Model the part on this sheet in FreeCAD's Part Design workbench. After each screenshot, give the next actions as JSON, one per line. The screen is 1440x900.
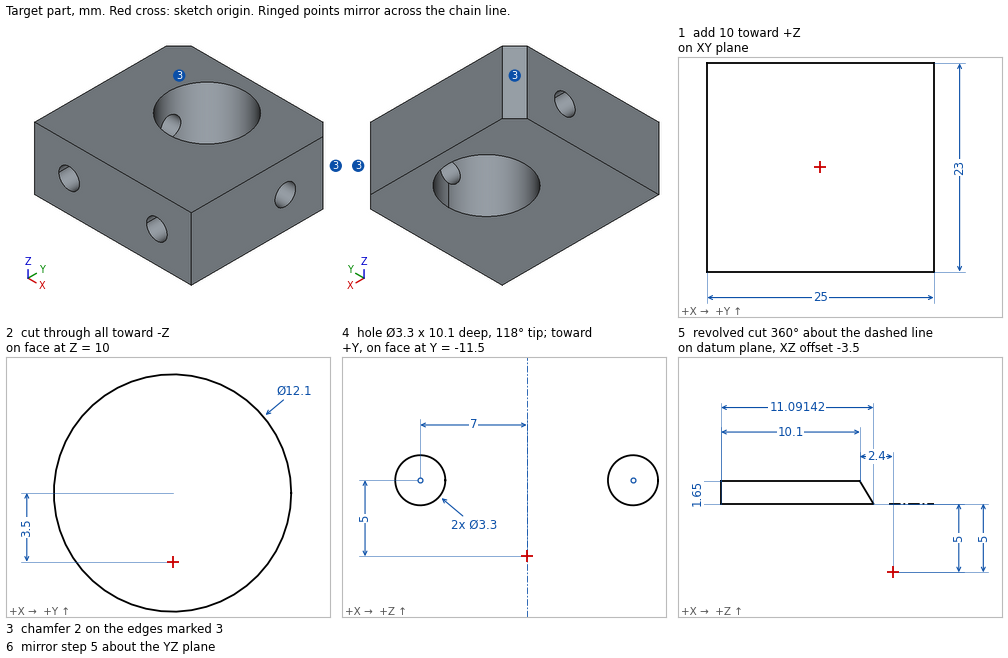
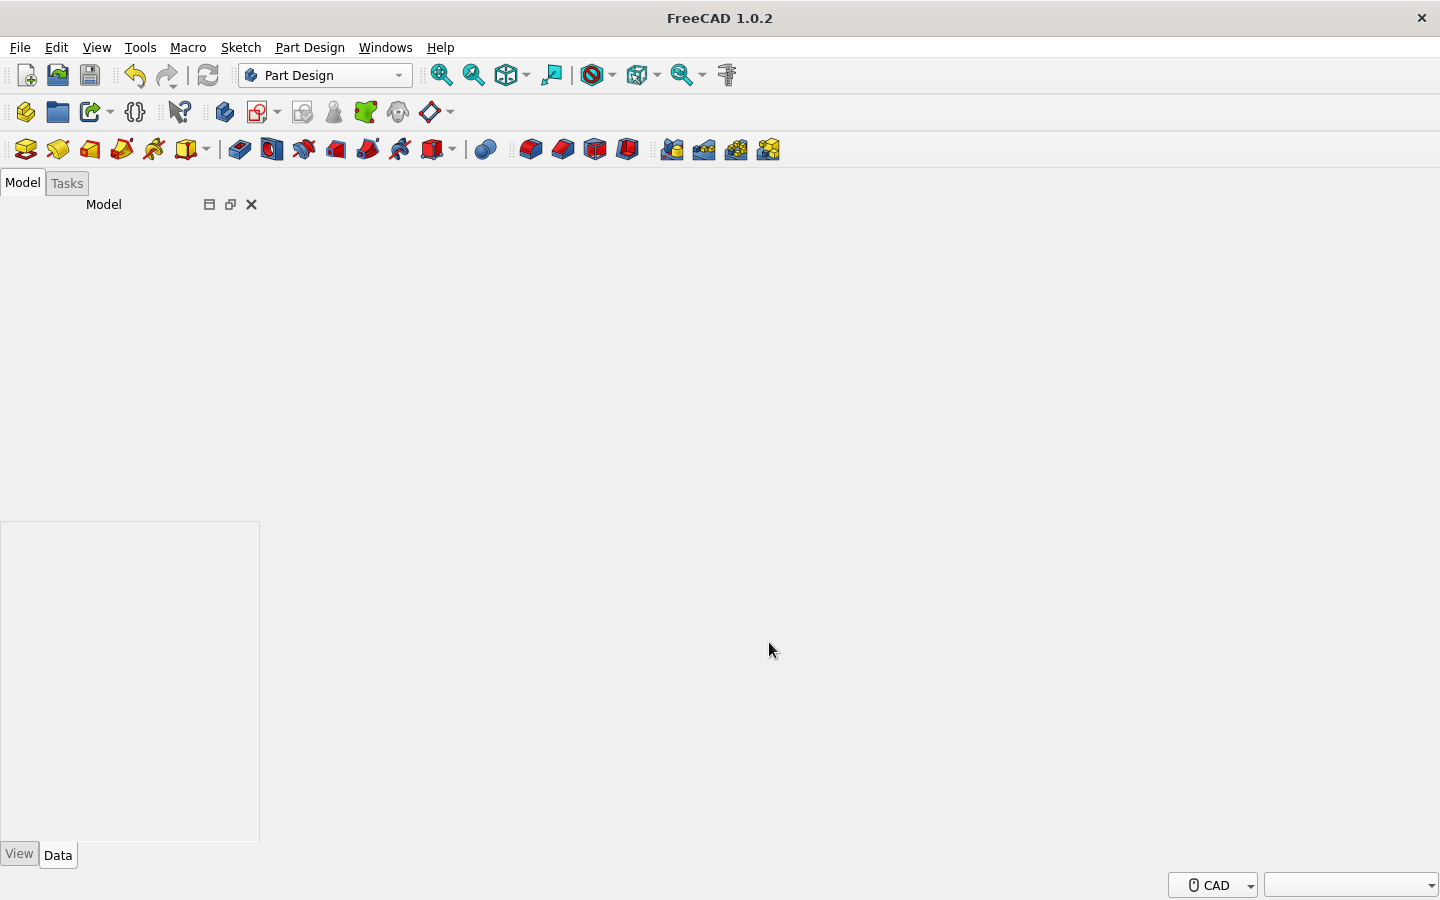
{"action": "left_click", "coordinate": [26, 76]}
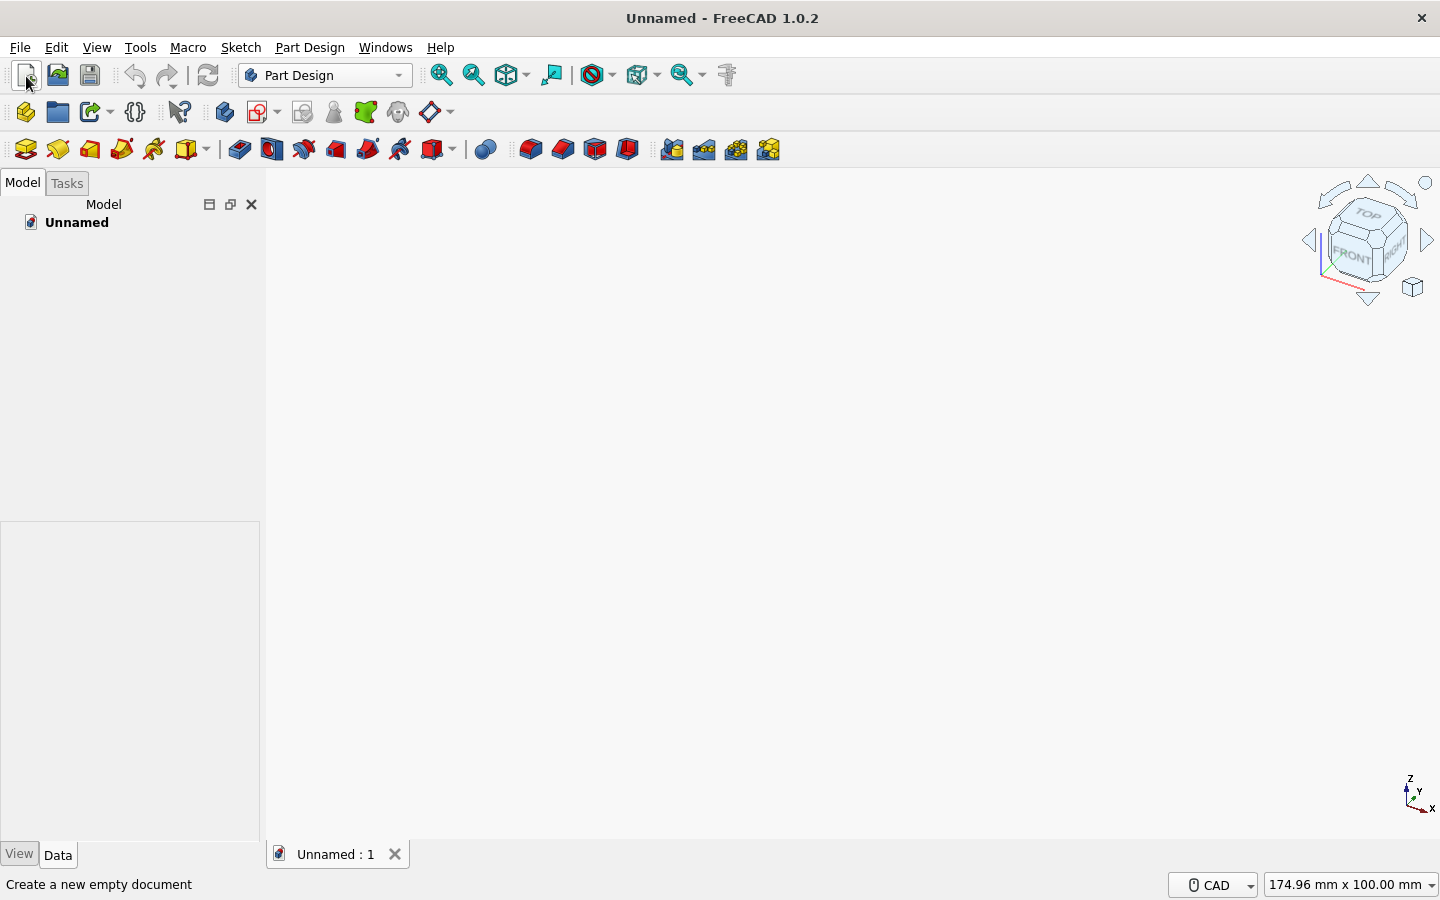
{"action": "left_click", "coordinate": [258, 112]}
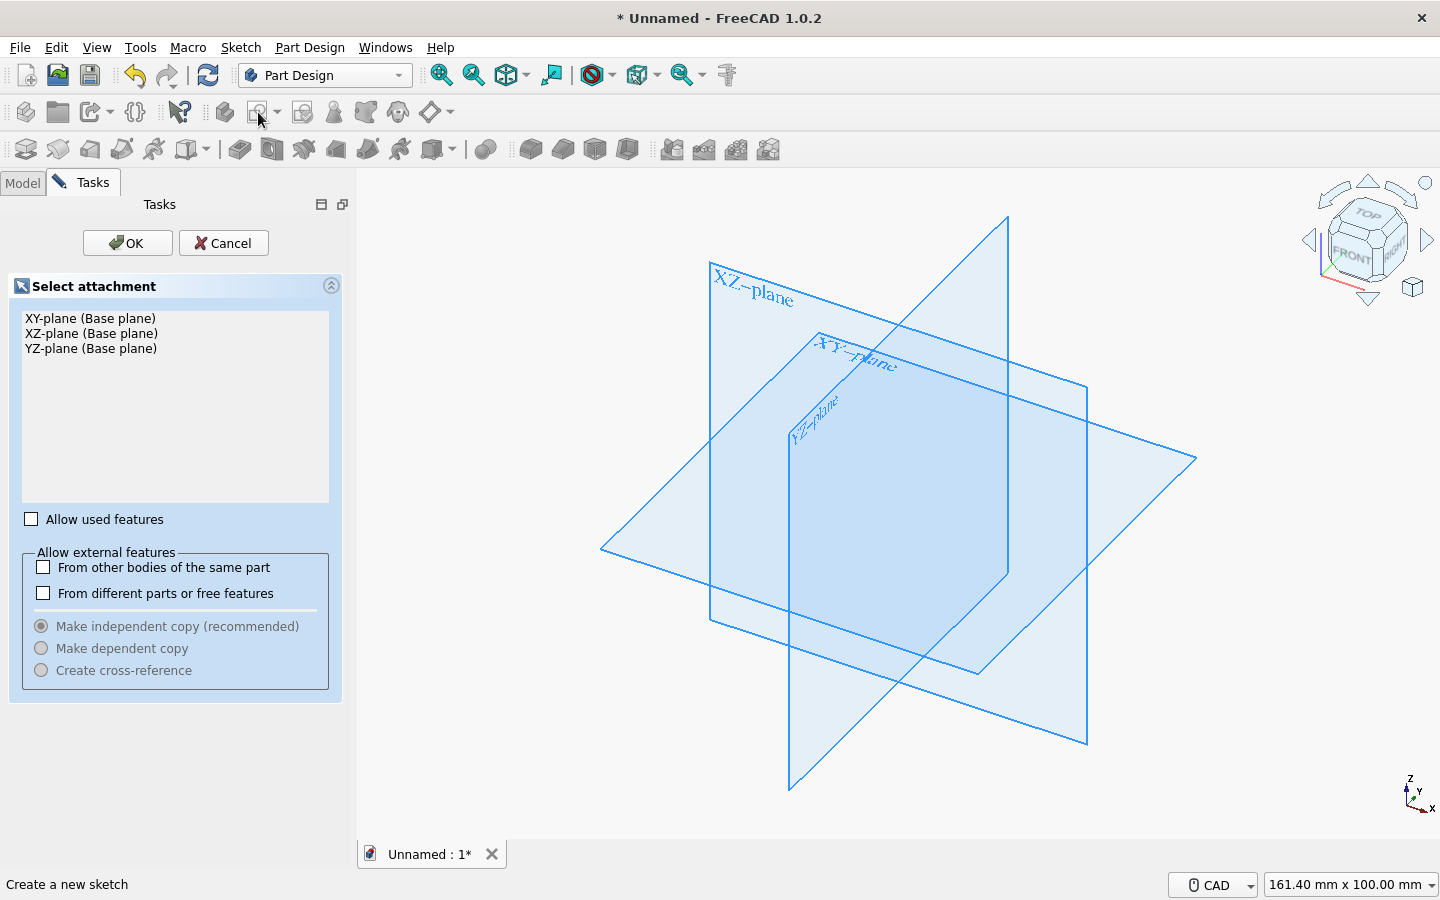
{"action": "left_click", "coordinate": [82, 318]}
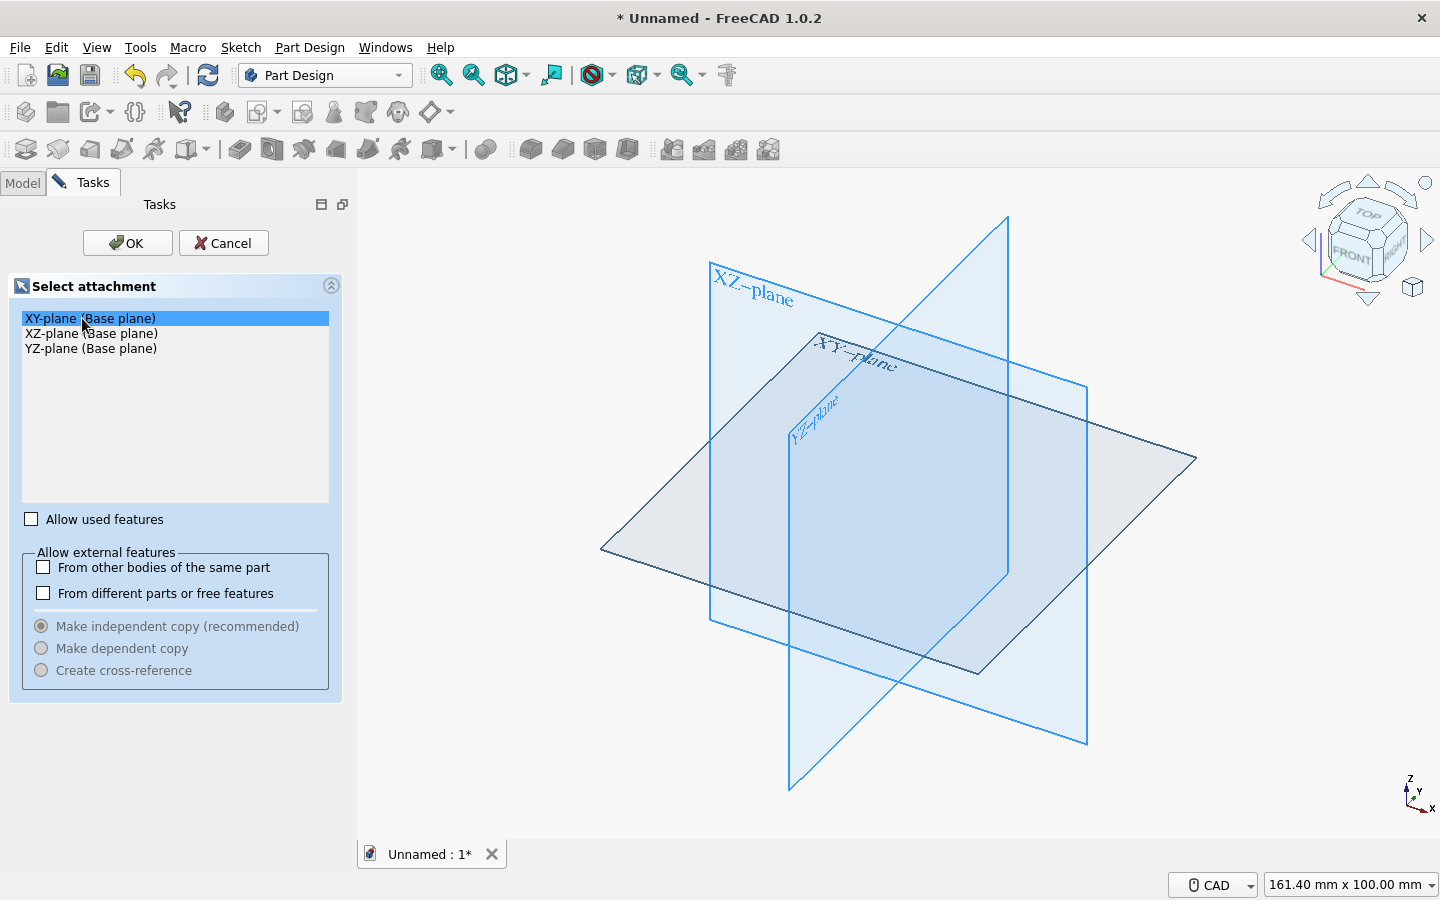
{"action": "left_click", "coordinate": [128, 243]}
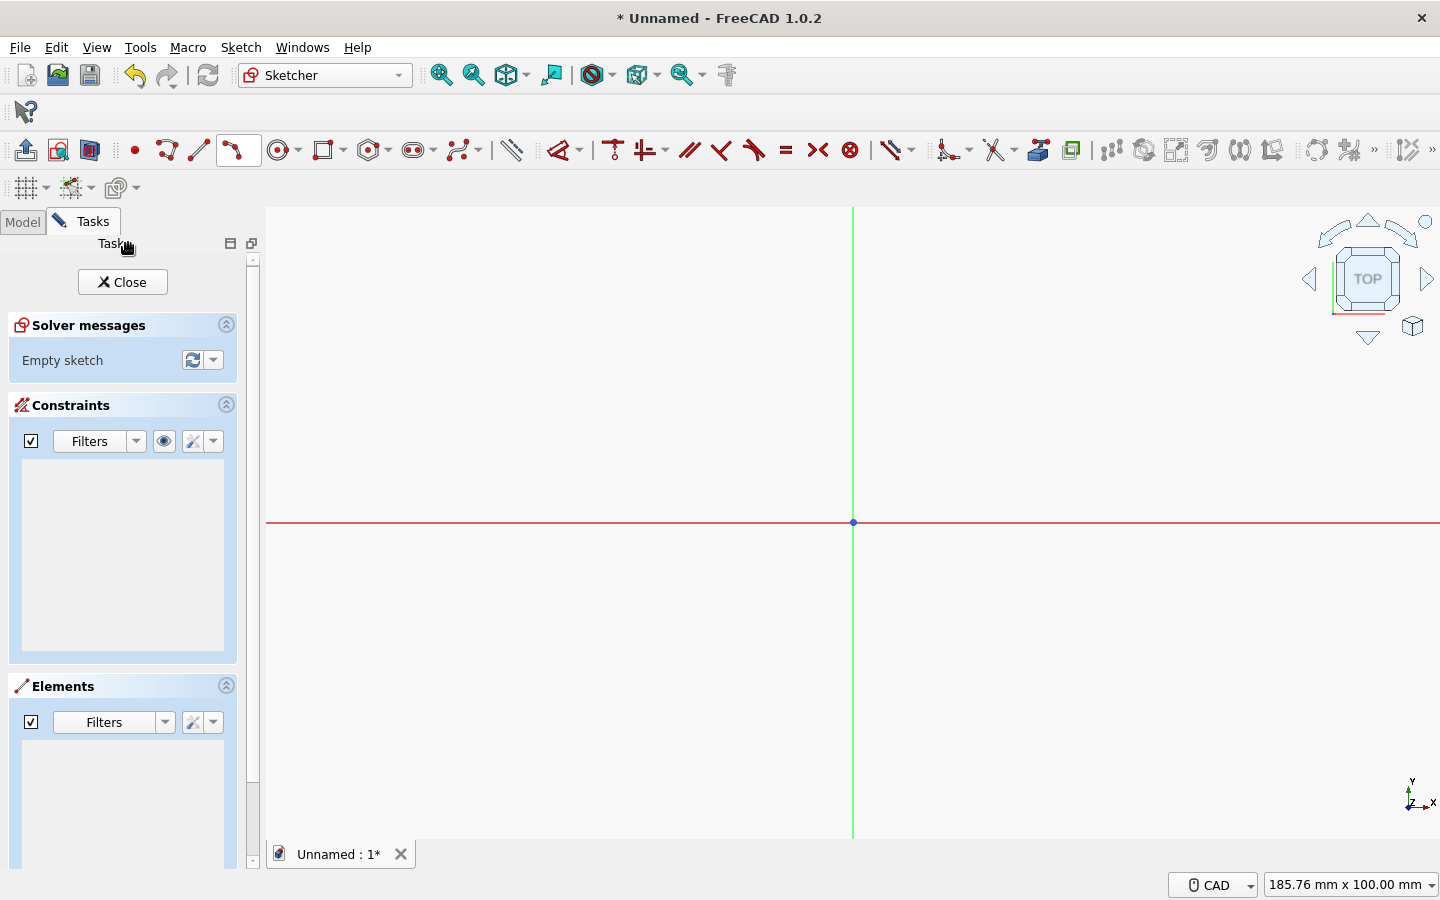
{"action": "scroll", "coordinate": [893, 523], "scroll_direction": "up", "scroll_amount": 5}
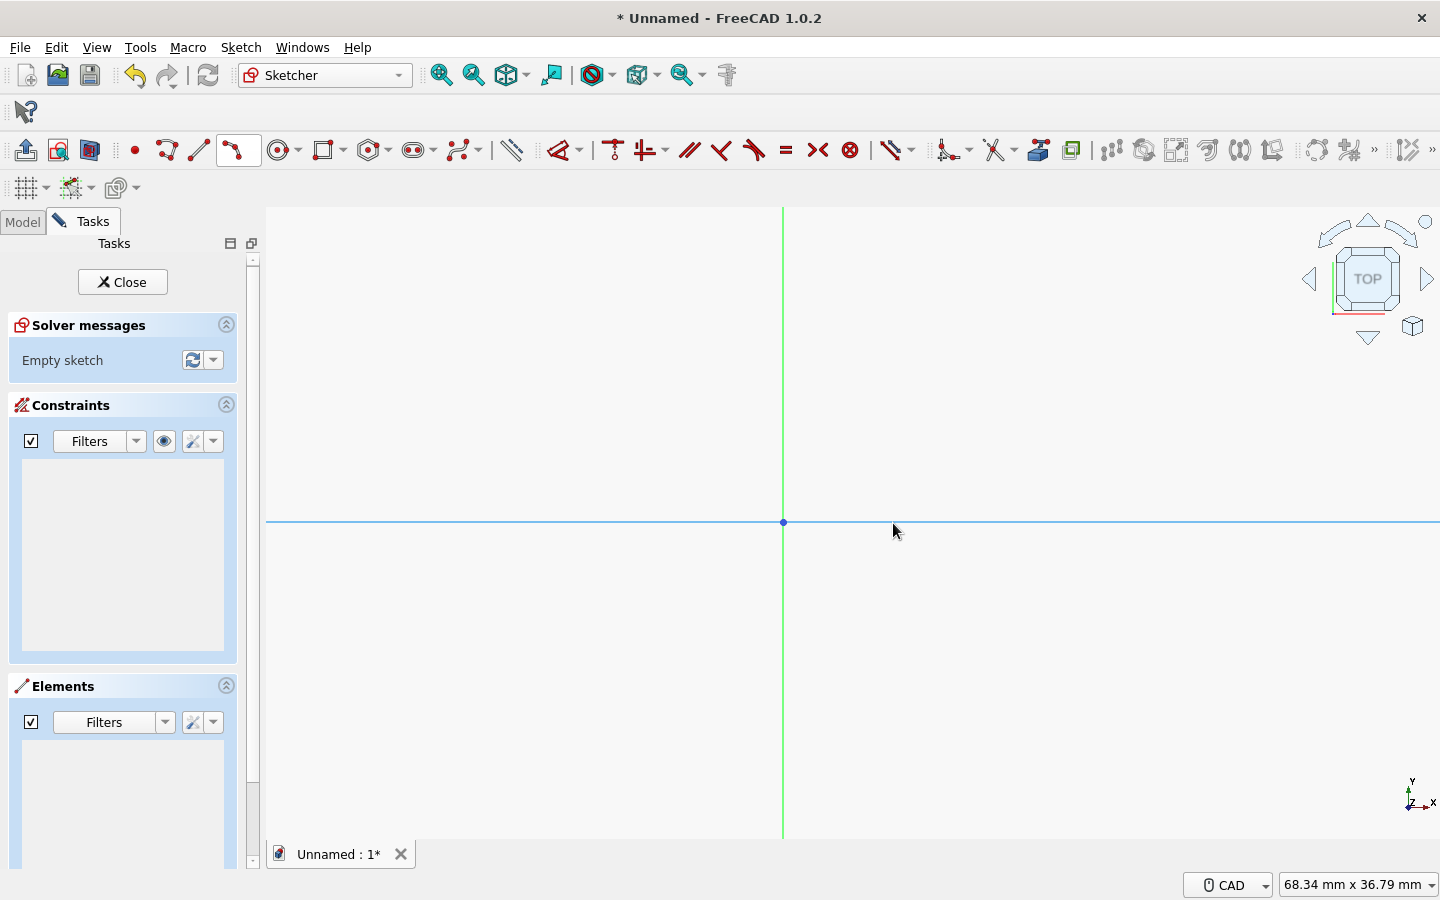
{"action": "key", "text": "g v"}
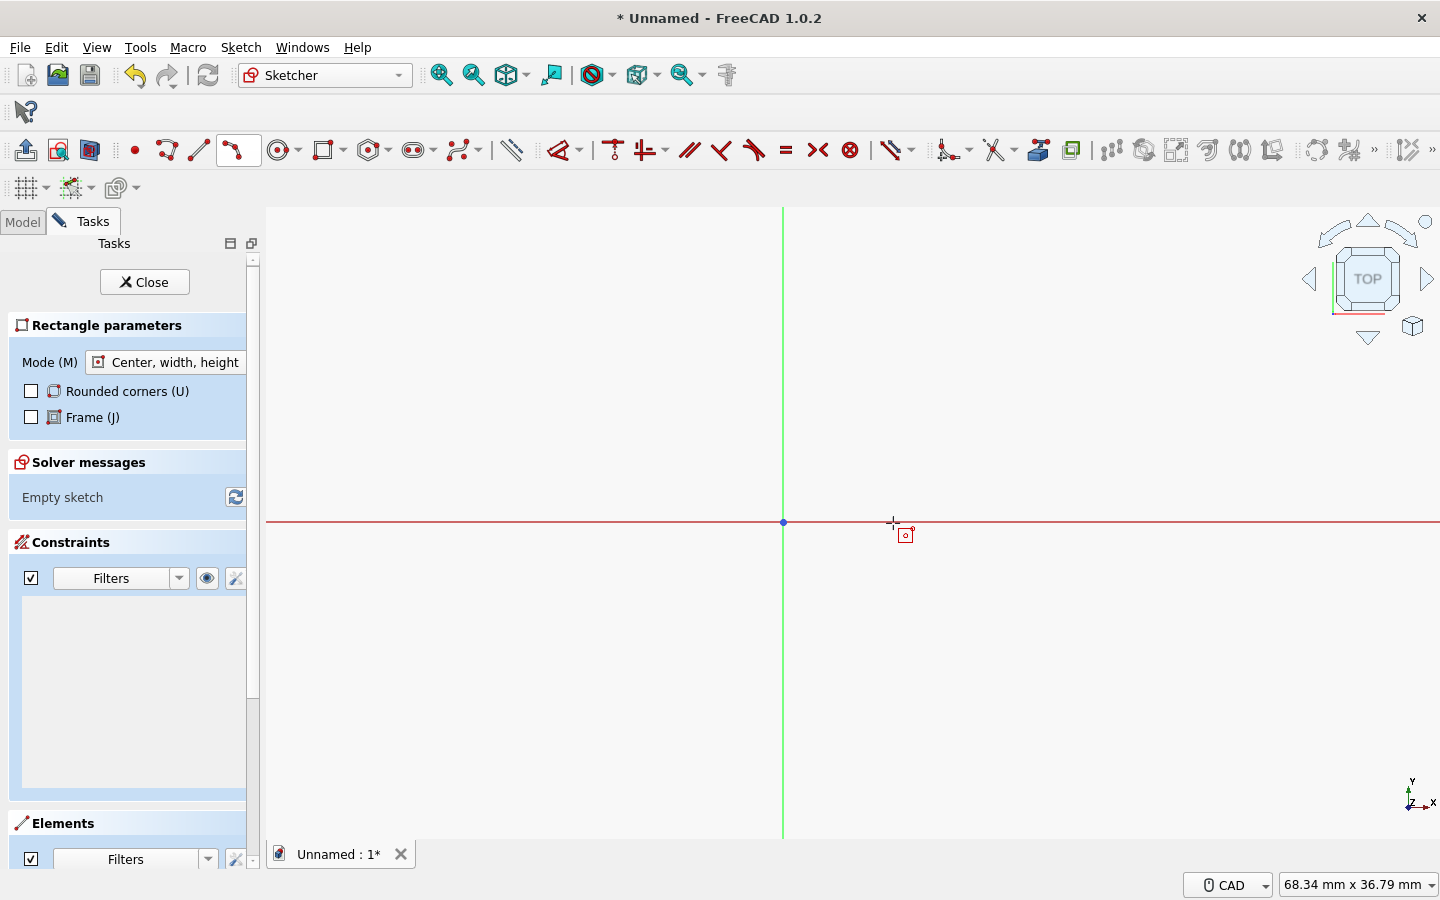
{"action": "left_click", "coordinate": [783, 522]}
{"action": "left_click", "coordinate": [998, 325]}
{"action": "key", "text": "Escape"}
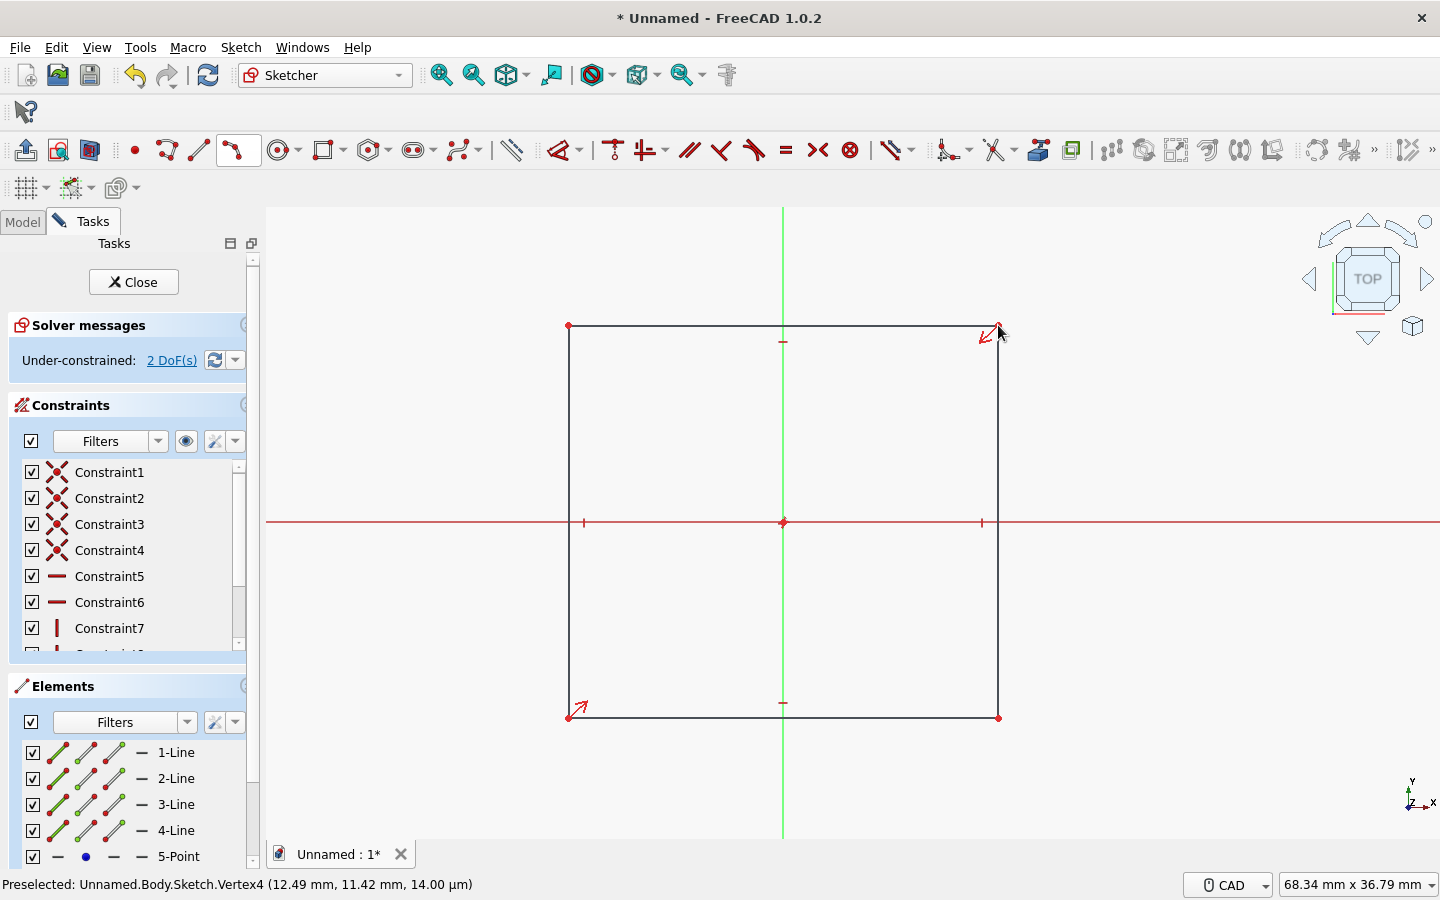
{"action": "key", "text": "d"}